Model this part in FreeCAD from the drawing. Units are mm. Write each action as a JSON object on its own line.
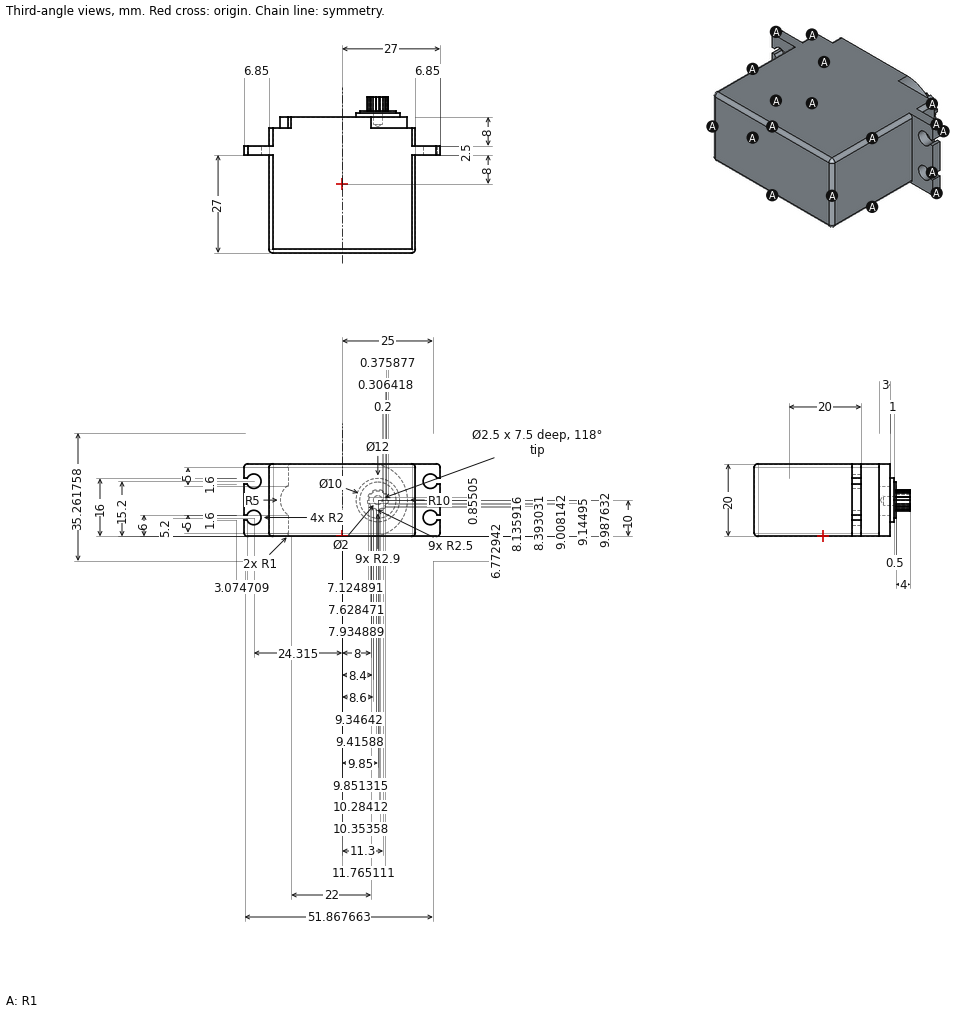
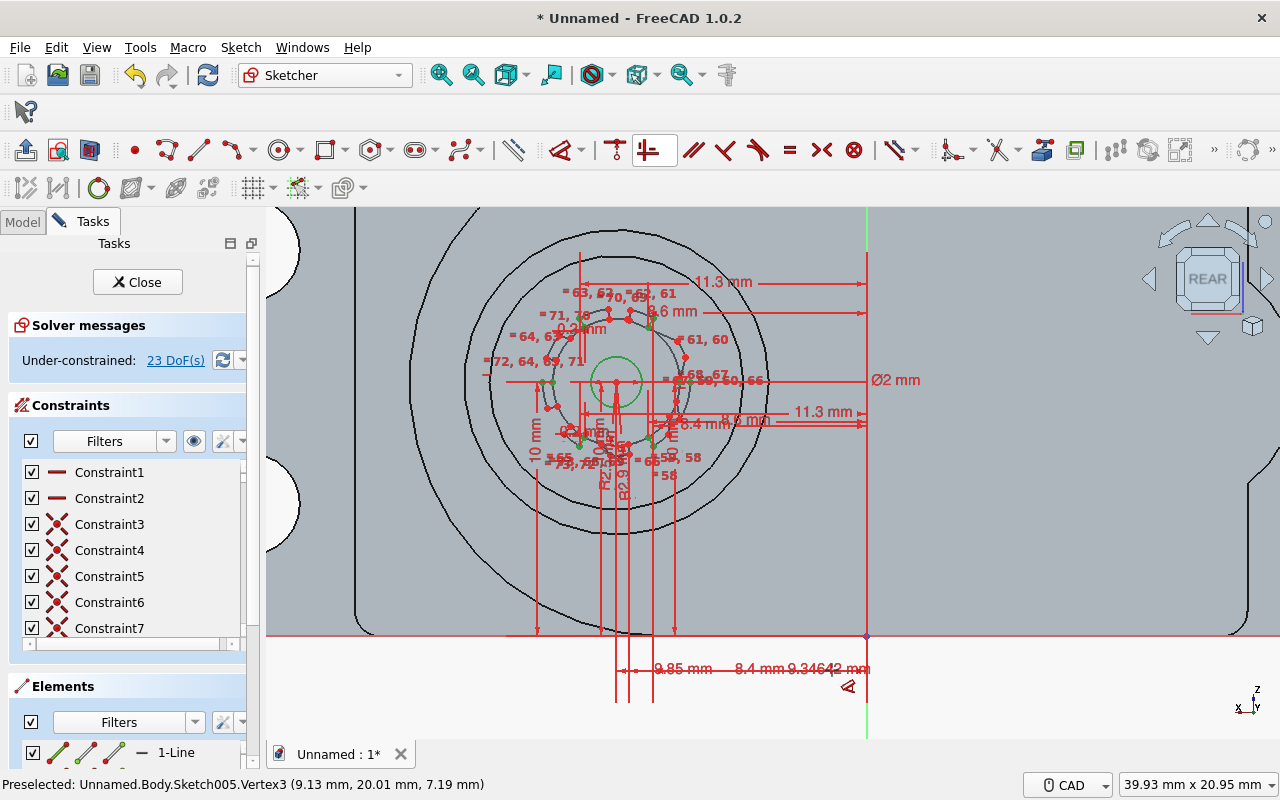
{"action": "left_click", "coordinate": [629, 445]}
{"action": "left_click", "coordinate": [748, 694]}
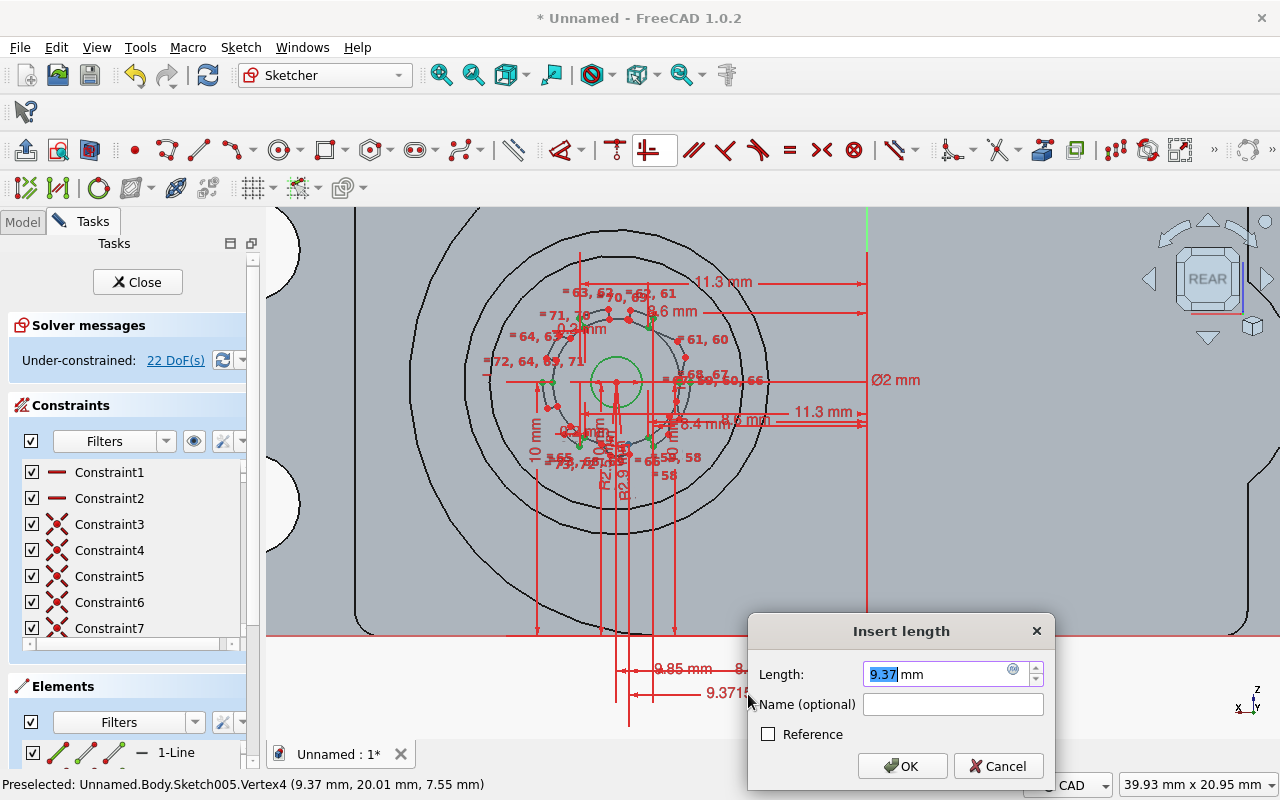
{"action": "type", "text": "9.41588"}
{"action": "key", "text": "Return"}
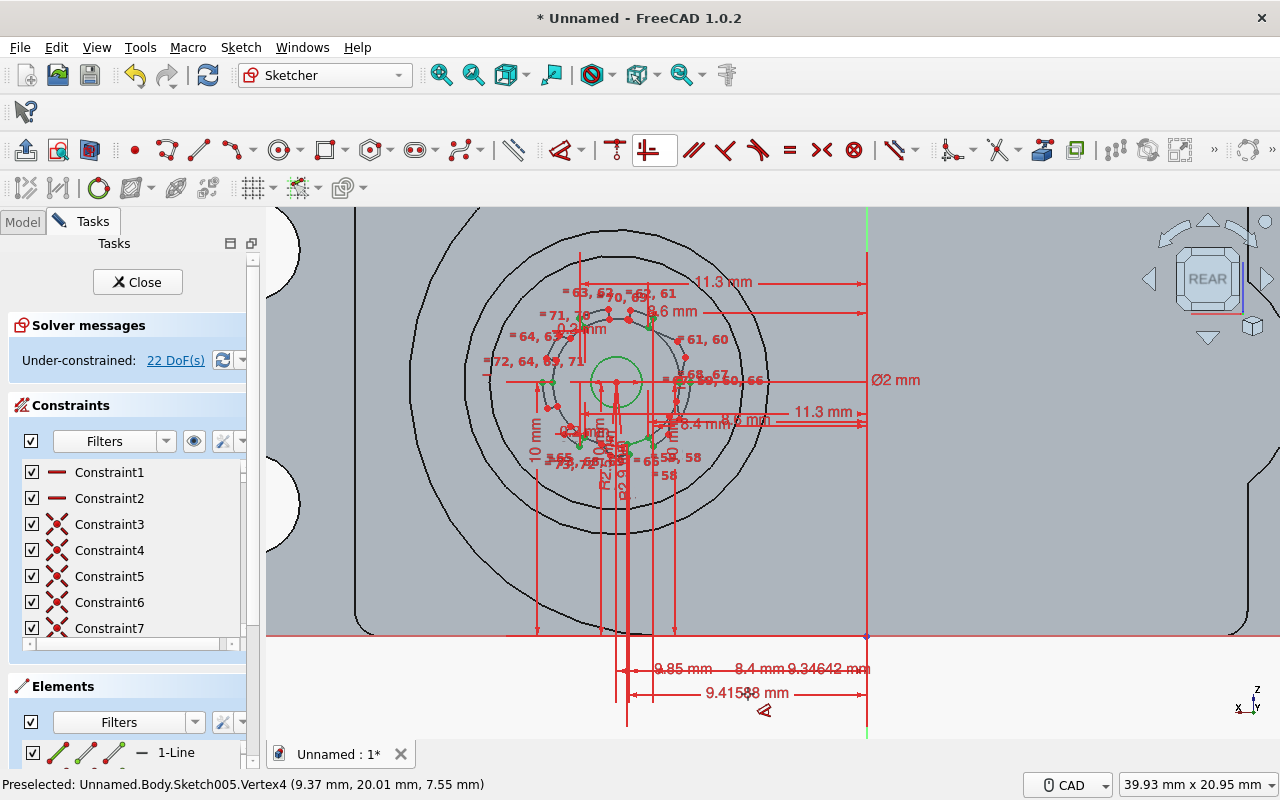
{"action": "left_click", "coordinate": [677, 402]}
{"action": "left_click", "coordinate": [901, 519]}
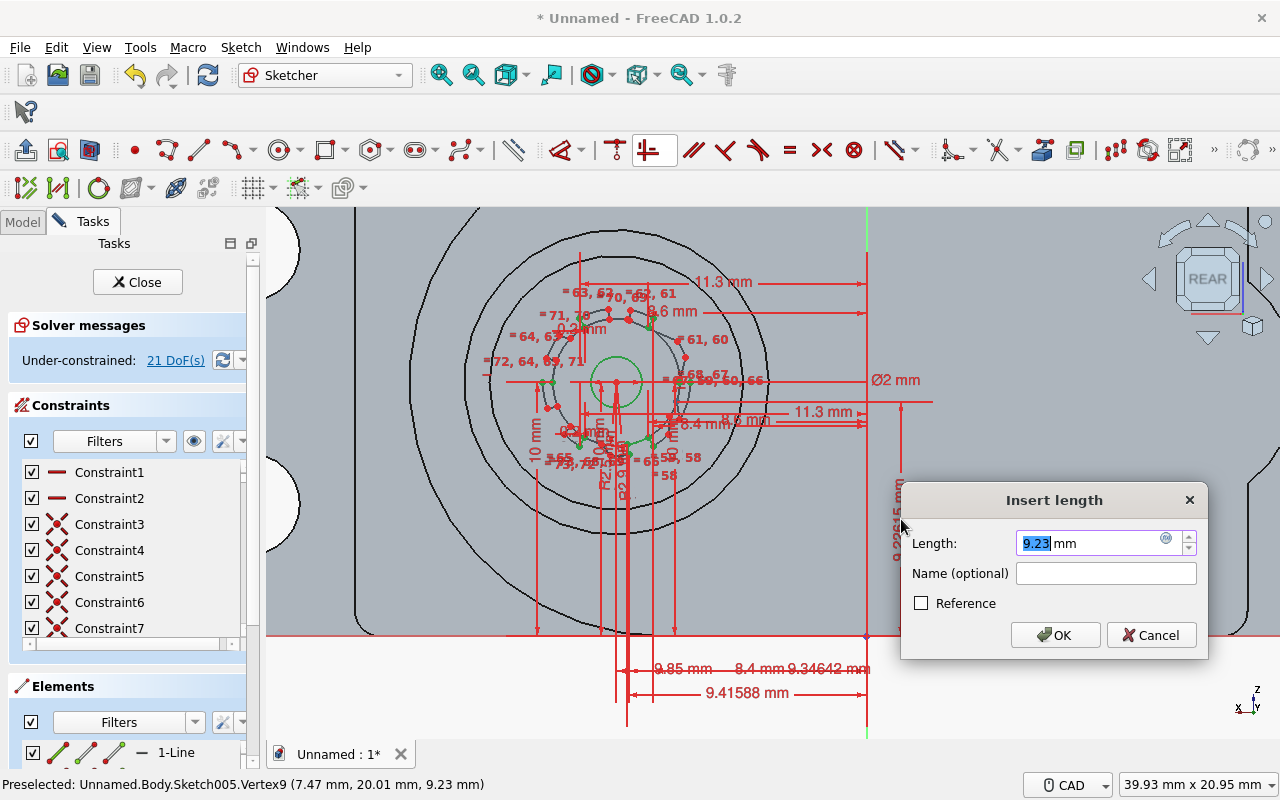
{"action": "type", "text": "9.14495"}
{"action": "key", "text": "Return"}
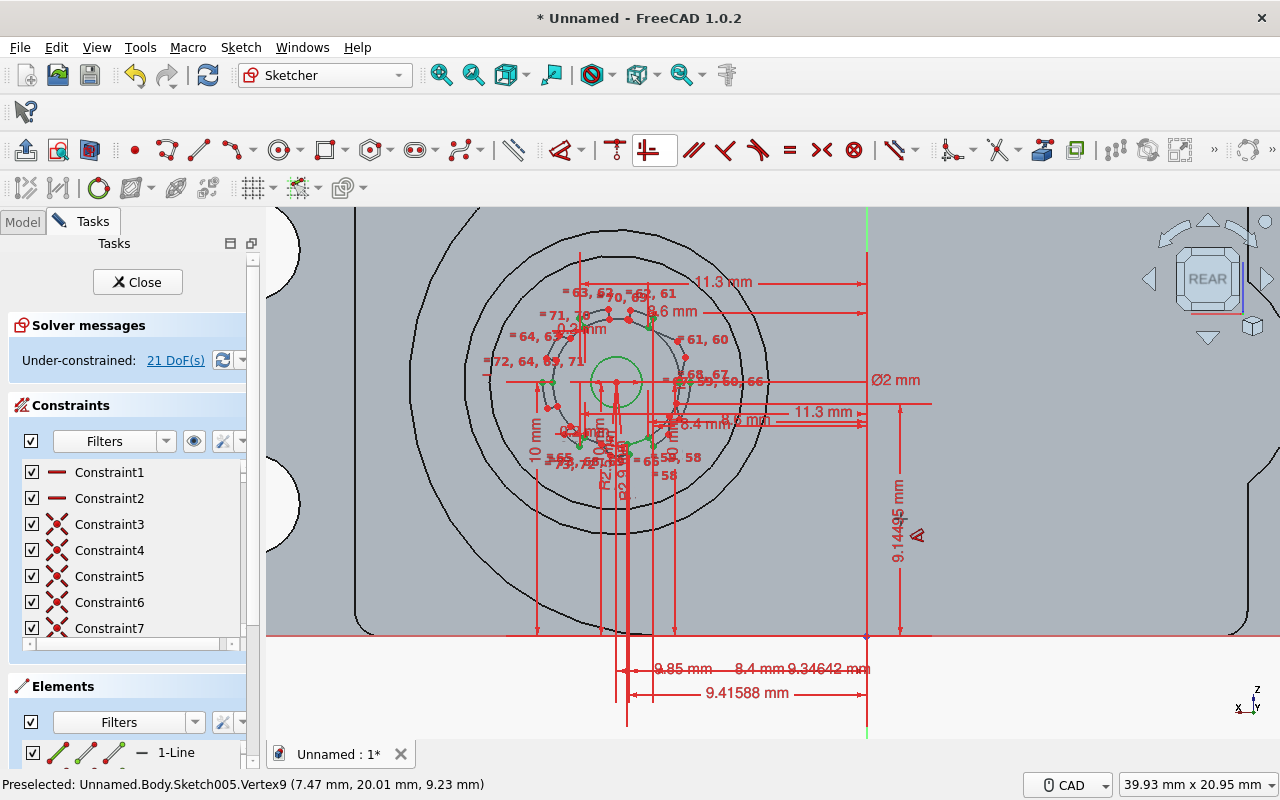
{"action": "left_click", "coordinate": [631, 310]}
{"action": "left_click", "coordinate": [803, 276]}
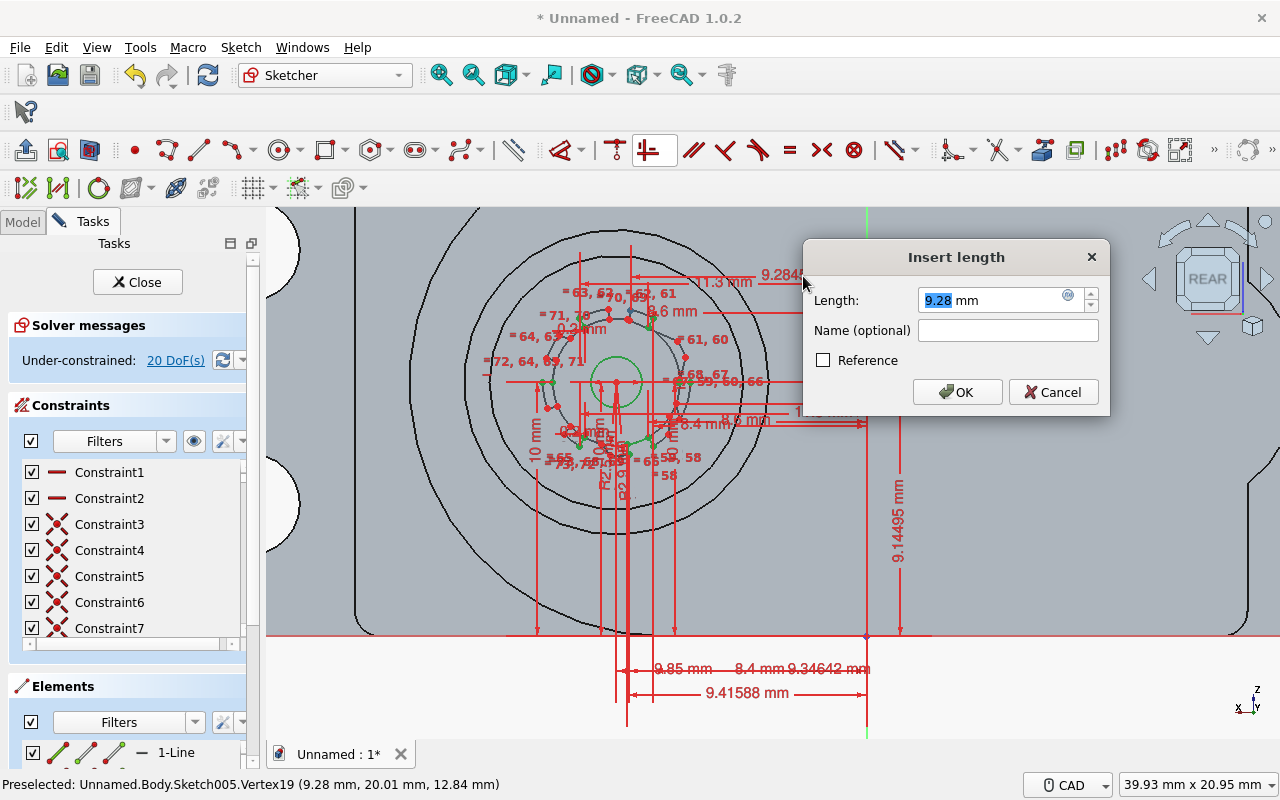
{"action": "type", "text": "9.34642"}
{"action": "key", "text": "Return"}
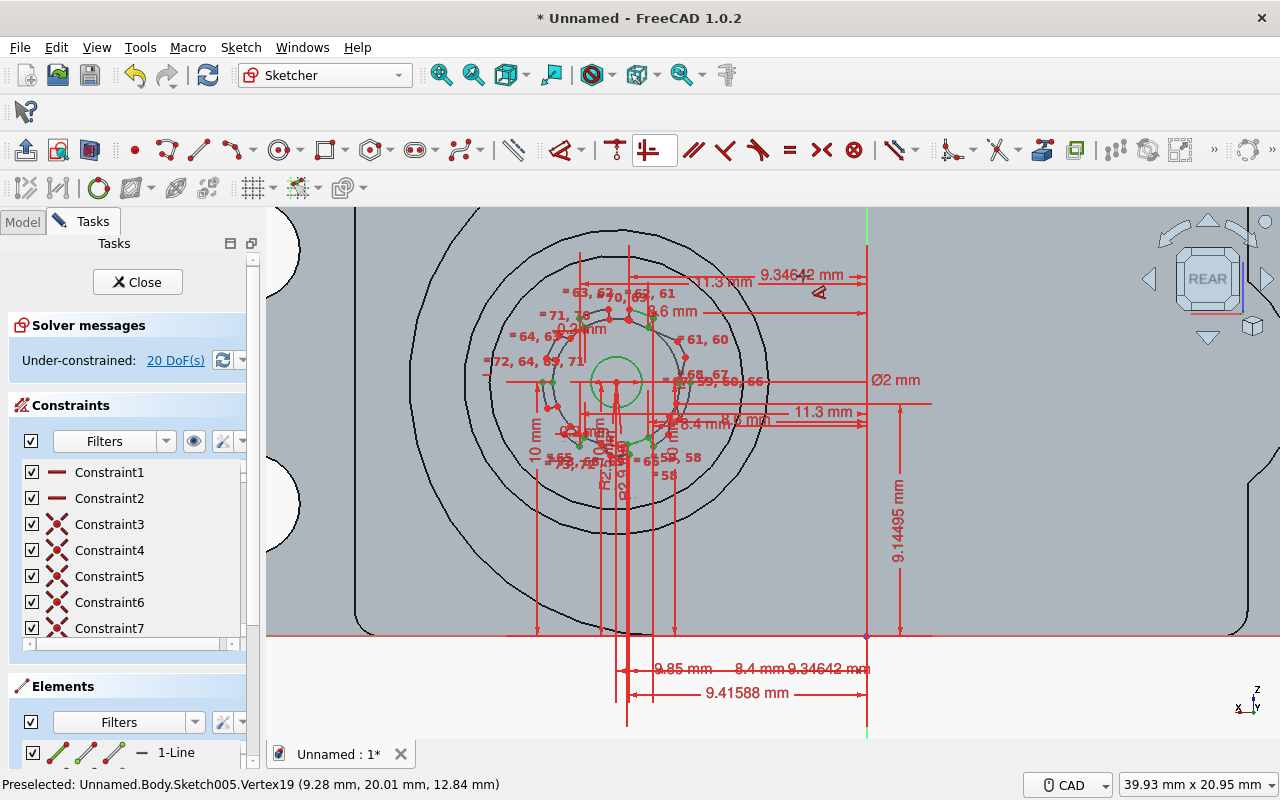
{"action": "scroll", "coordinate": [630, 320], "scroll_direction": "up", "scroll_amount": 10}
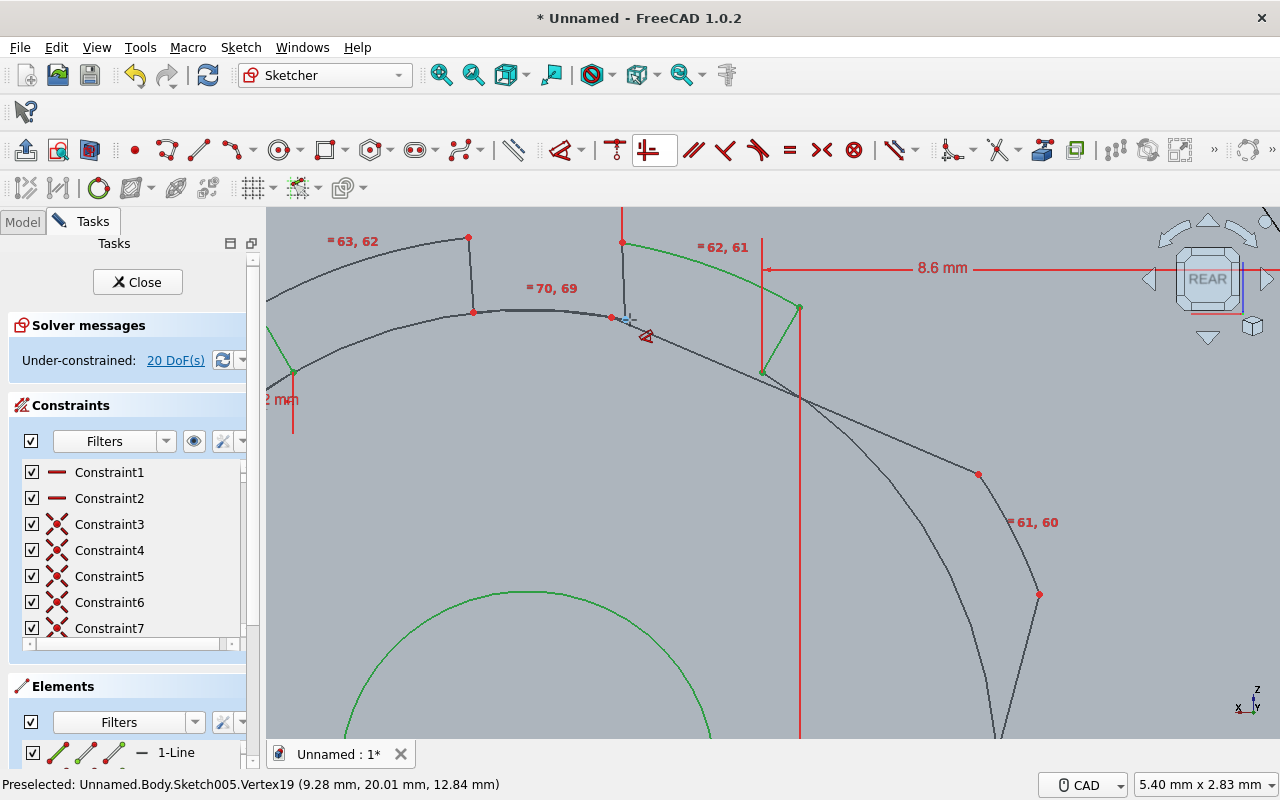
{"action": "left_click", "coordinate": [625, 320]}
{"action": "left_click", "coordinate": [983, 286]}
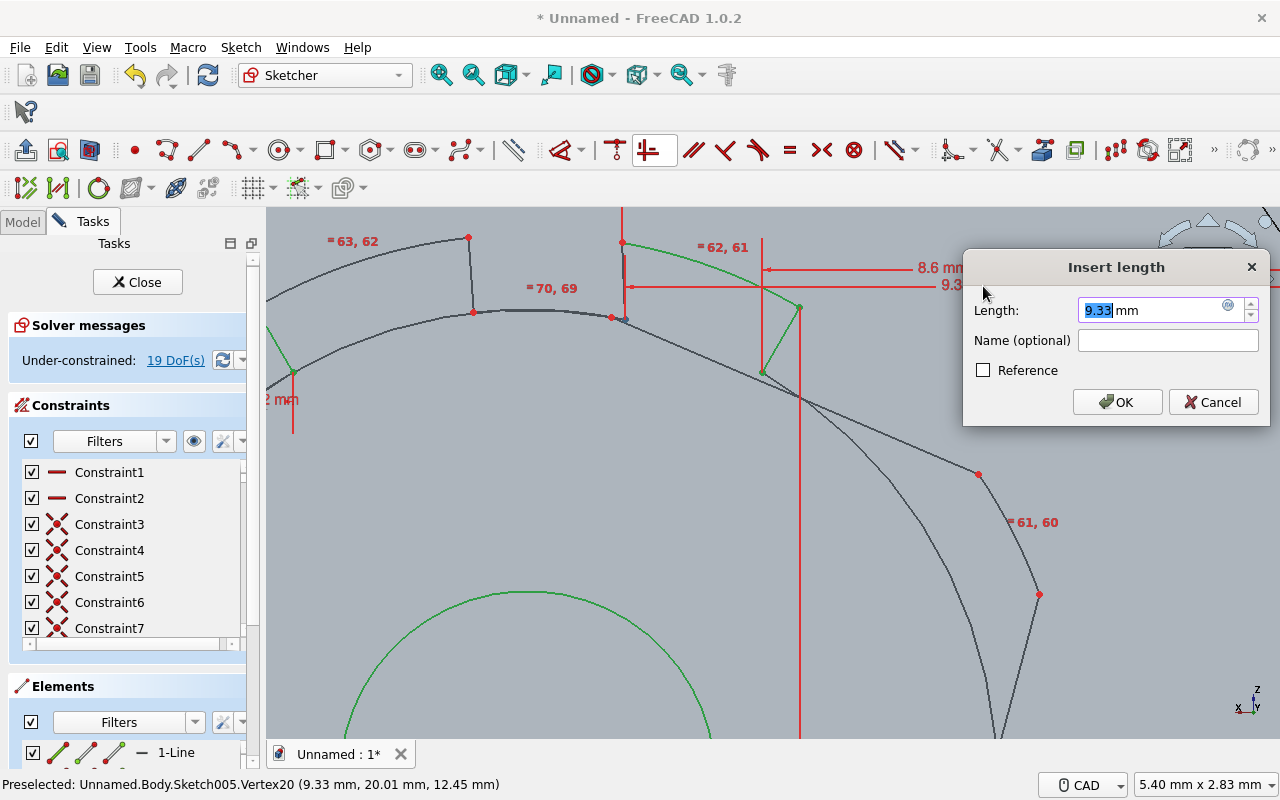
{"action": "type", "text": "9.41588"}
{"action": "key", "text": "Return"}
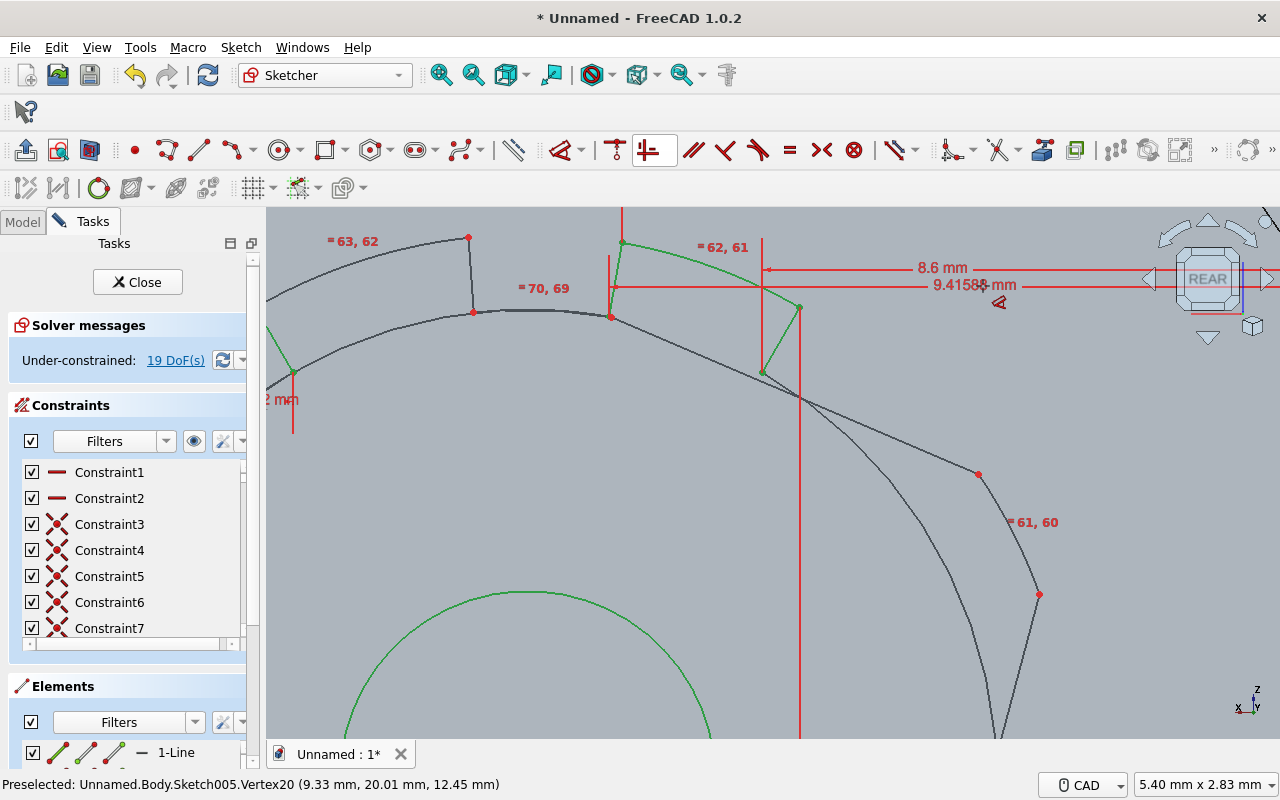
{"action": "scroll", "coordinate": [630, 320], "scroll_direction": "down", "scroll_amount": 10}